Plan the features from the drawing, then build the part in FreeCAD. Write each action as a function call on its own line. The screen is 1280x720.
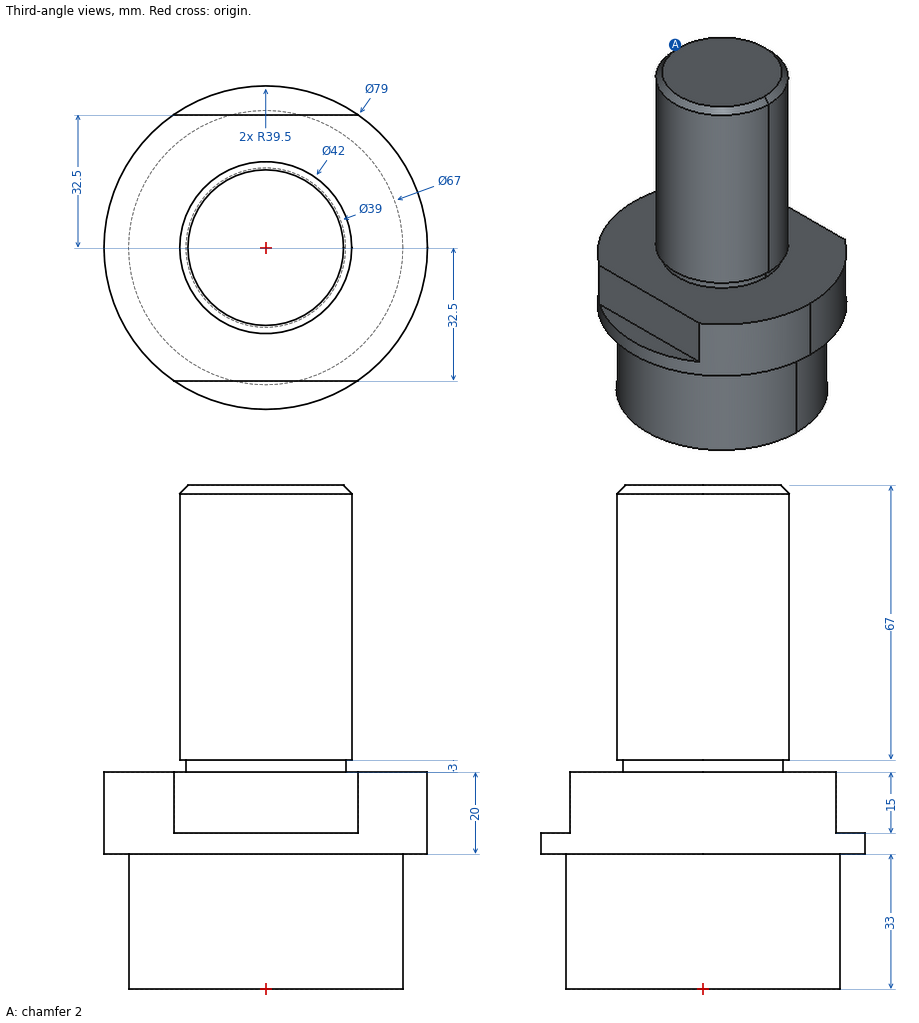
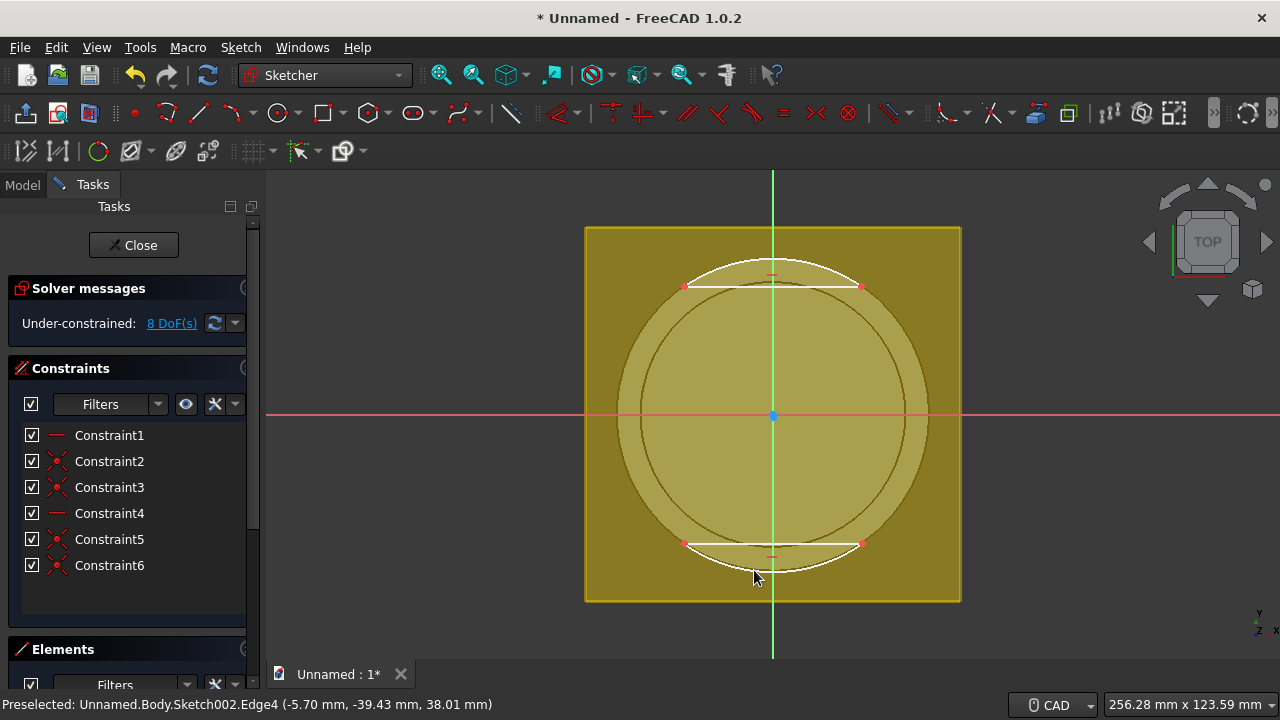
click(810, 263)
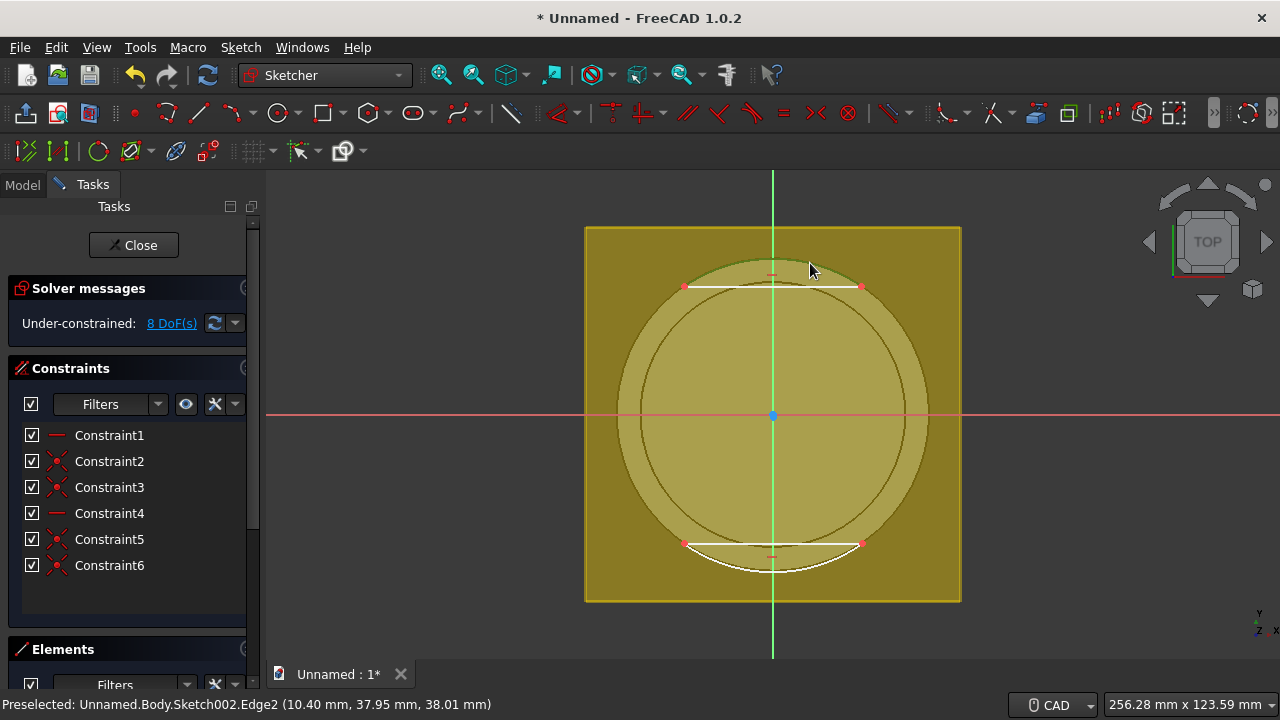
click(735, 568)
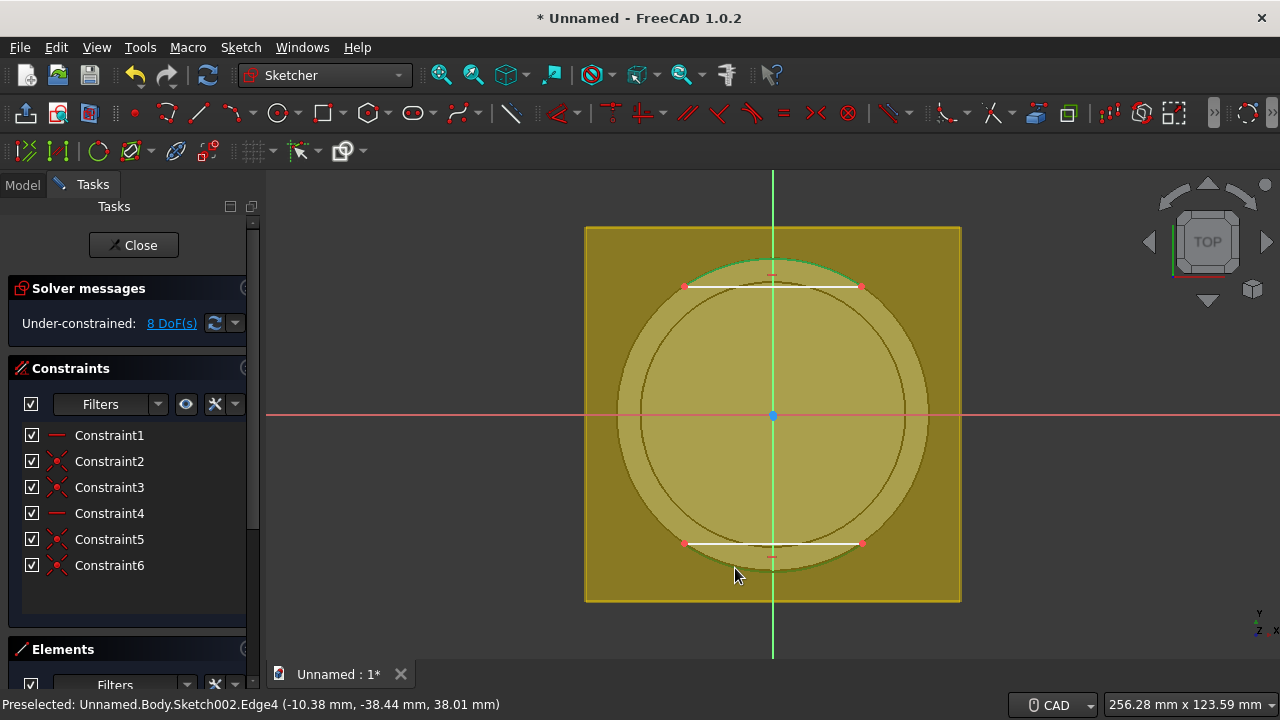
click(612, 114)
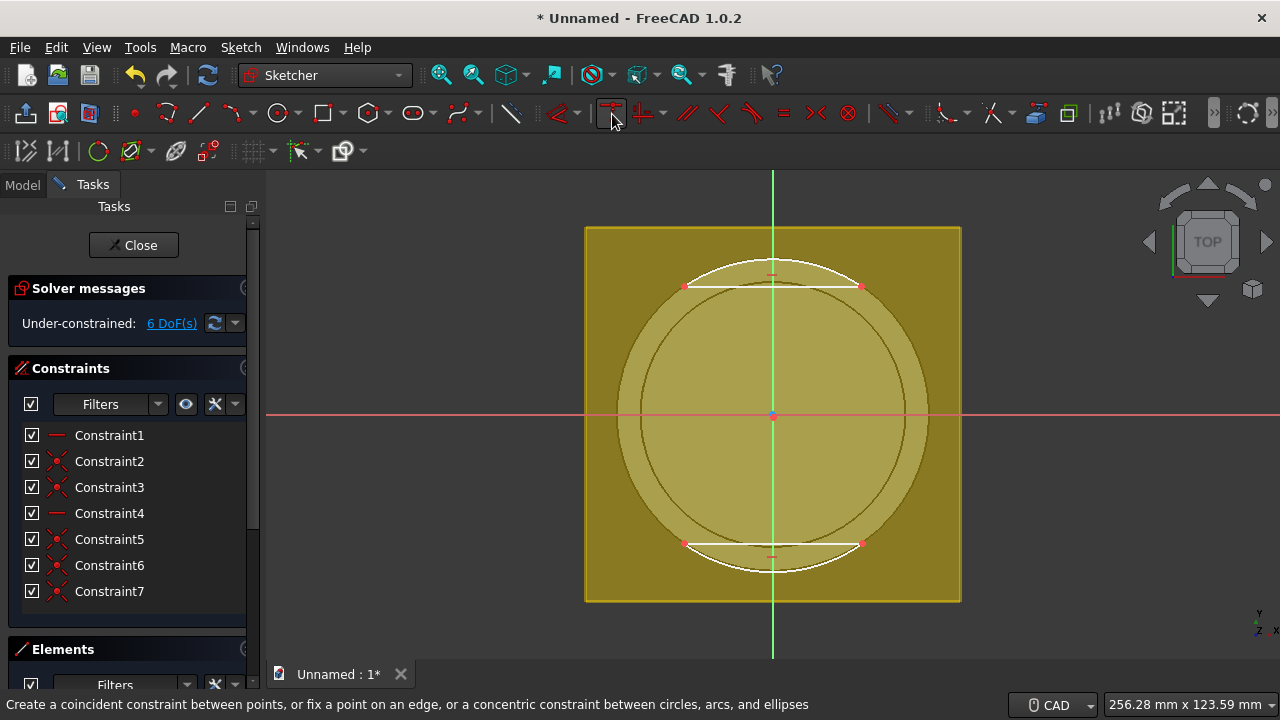
drag(763, 404, 783, 427)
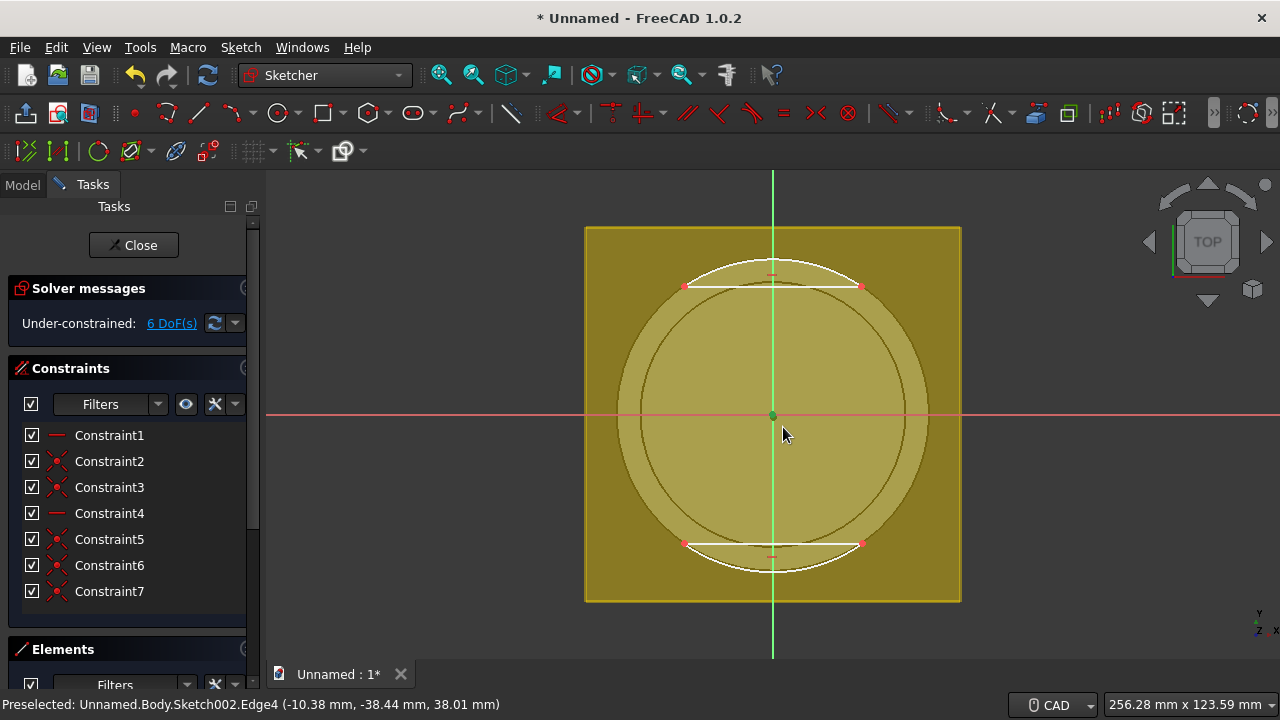
click(612, 114)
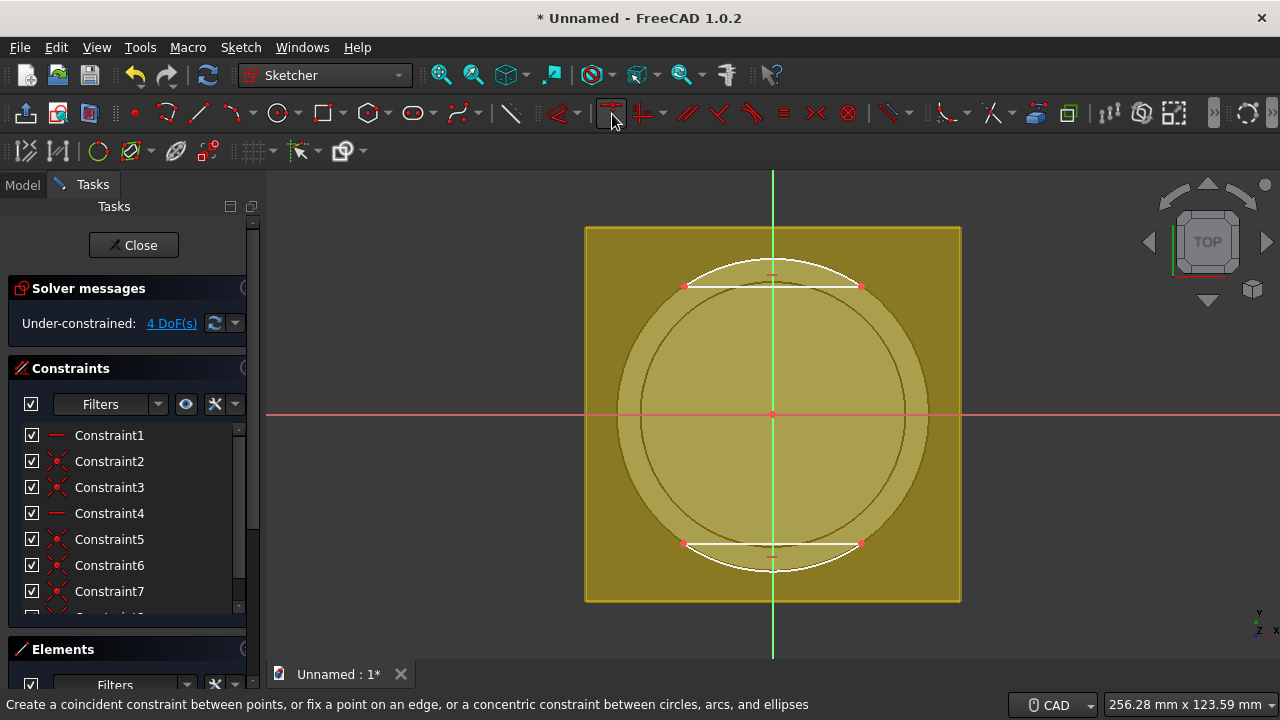
click(810, 263)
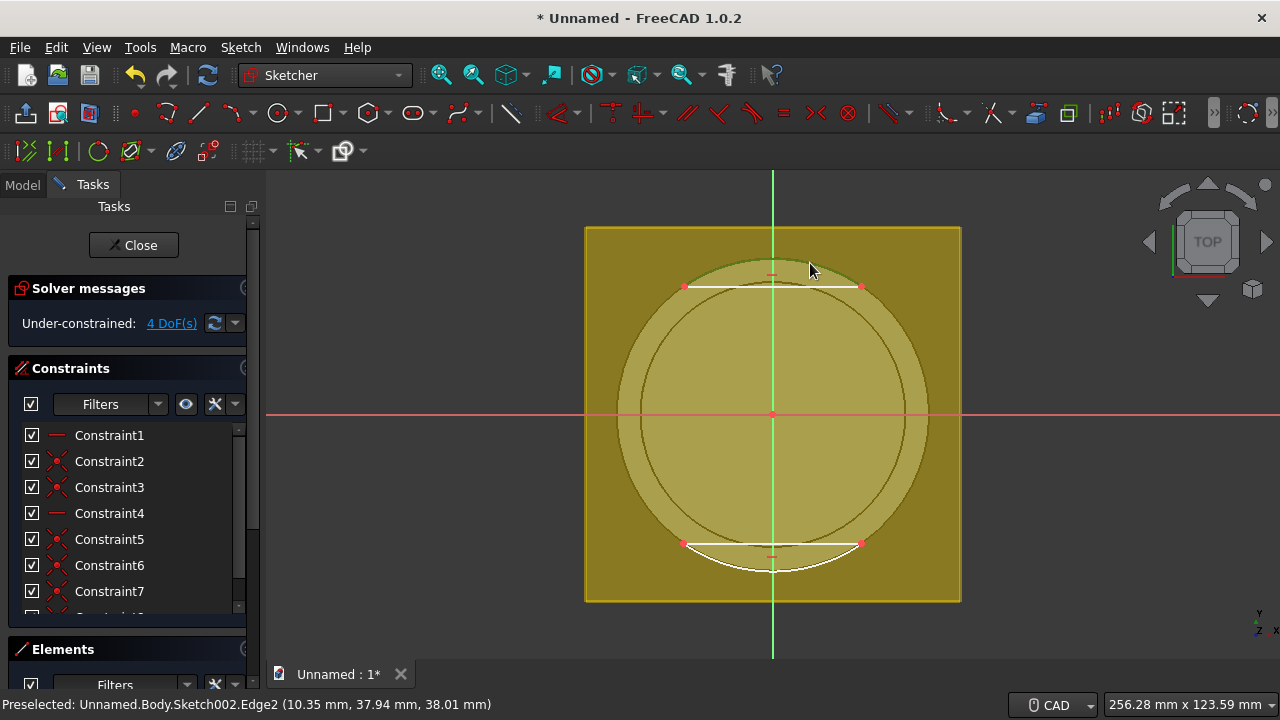
click(735, 567)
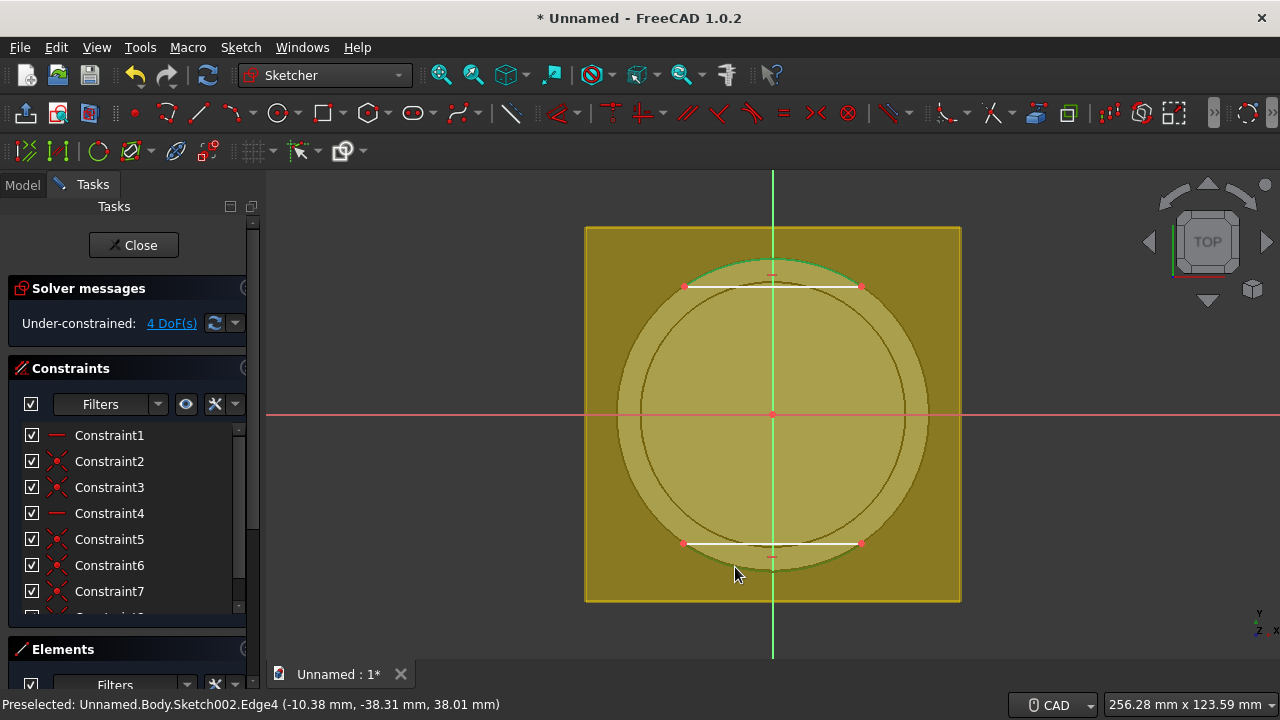
click(784, 114)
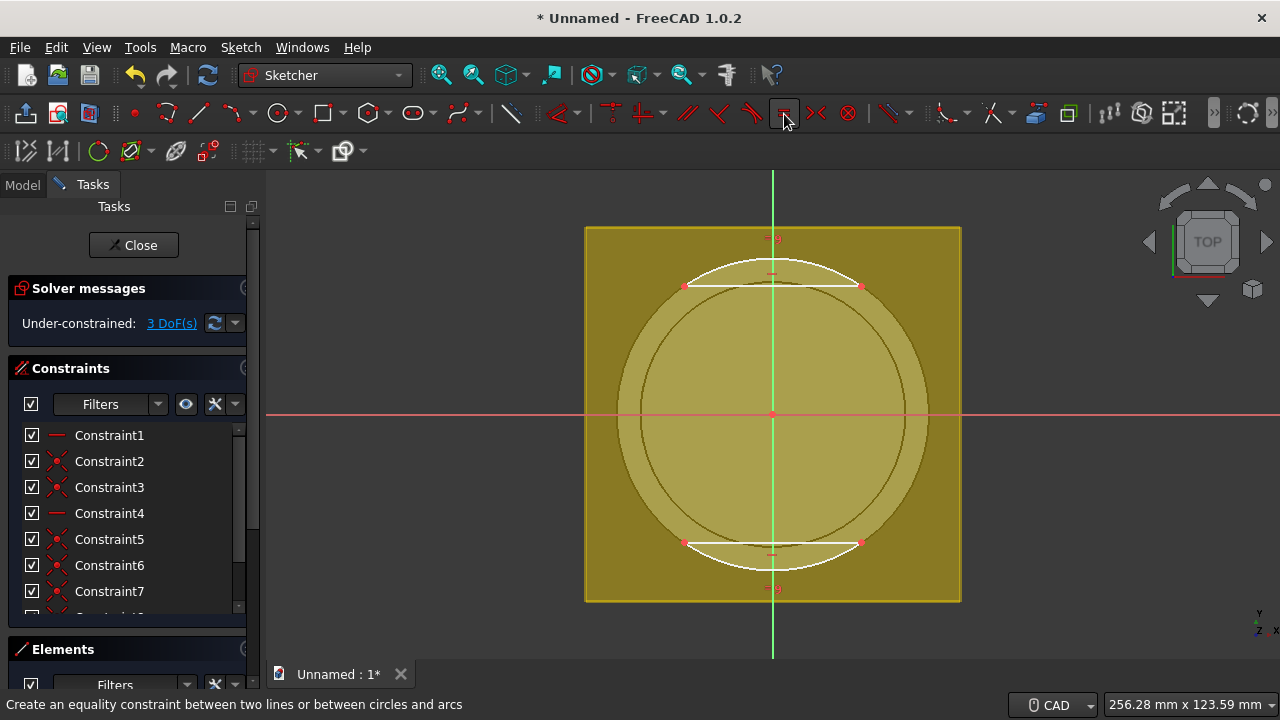
click(558, 114)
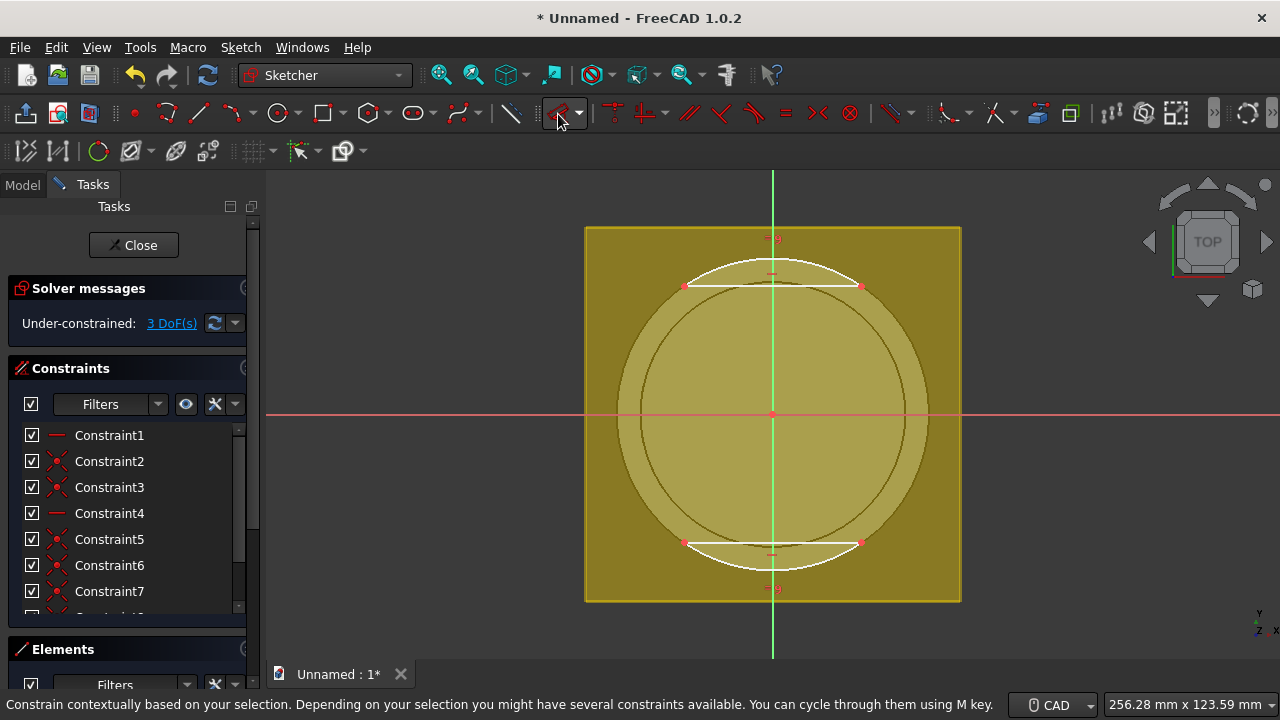
click(810, 263)
click(818, 232)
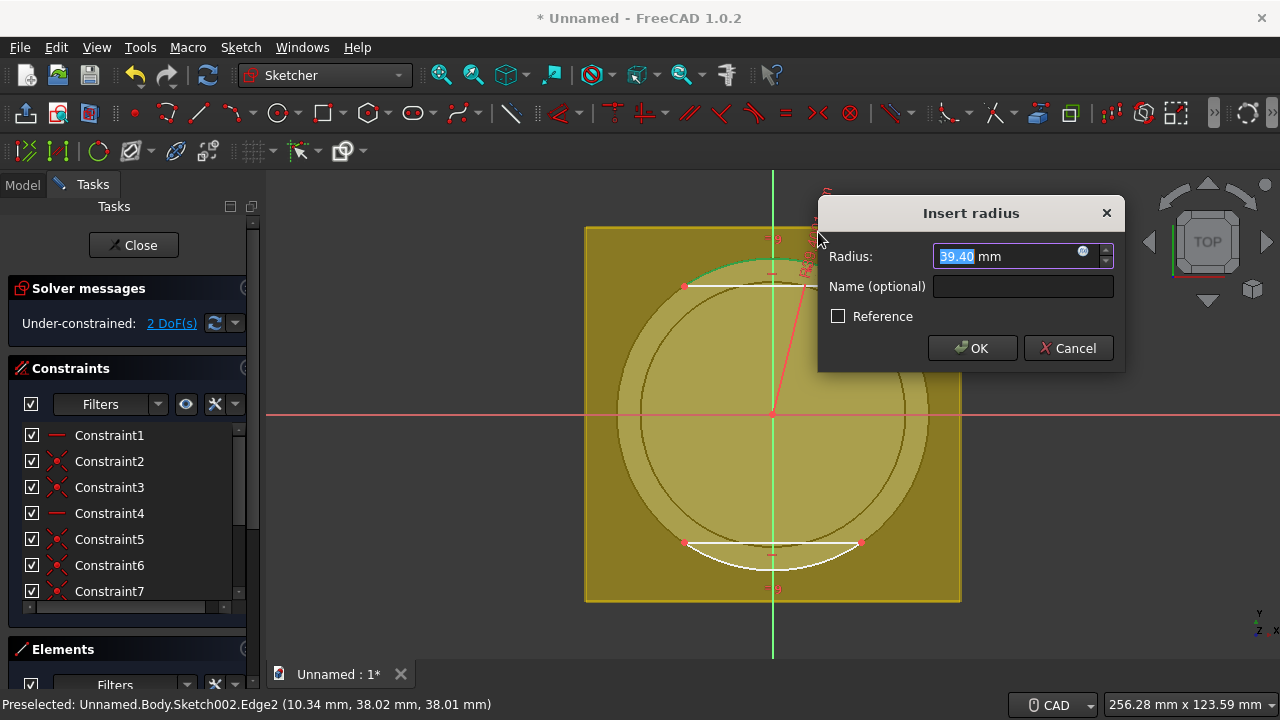
text(39.5)
key(Return)